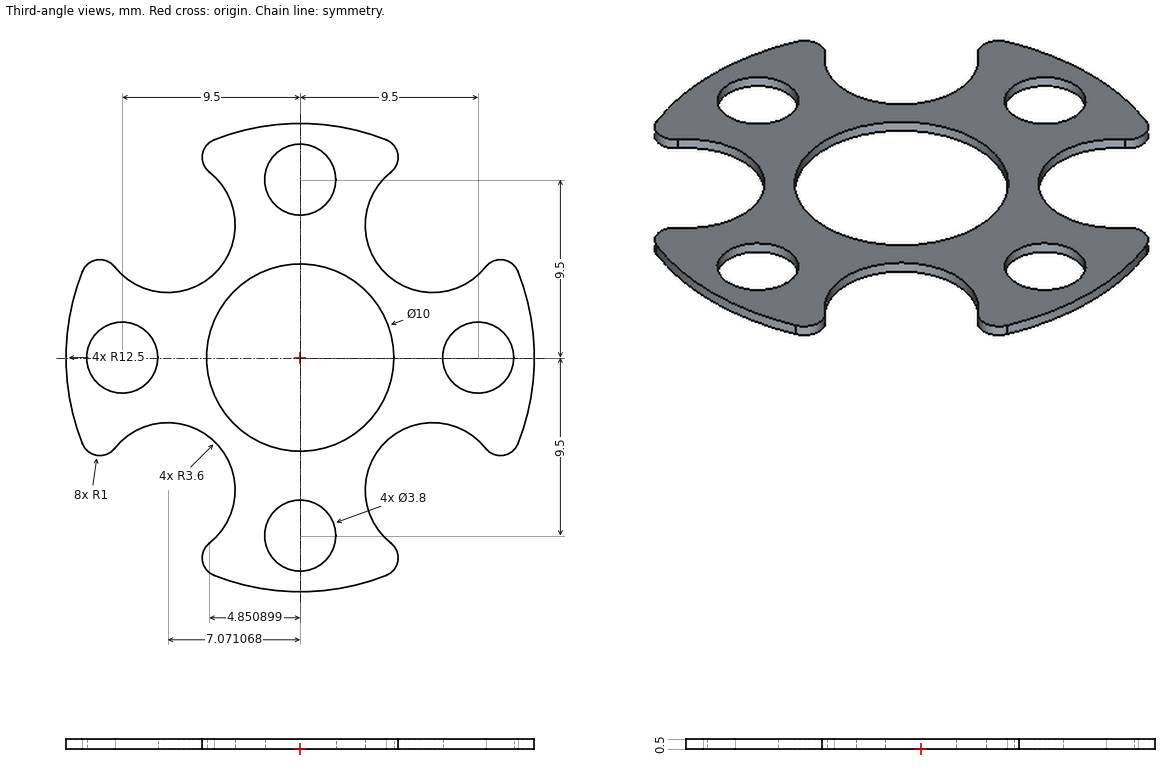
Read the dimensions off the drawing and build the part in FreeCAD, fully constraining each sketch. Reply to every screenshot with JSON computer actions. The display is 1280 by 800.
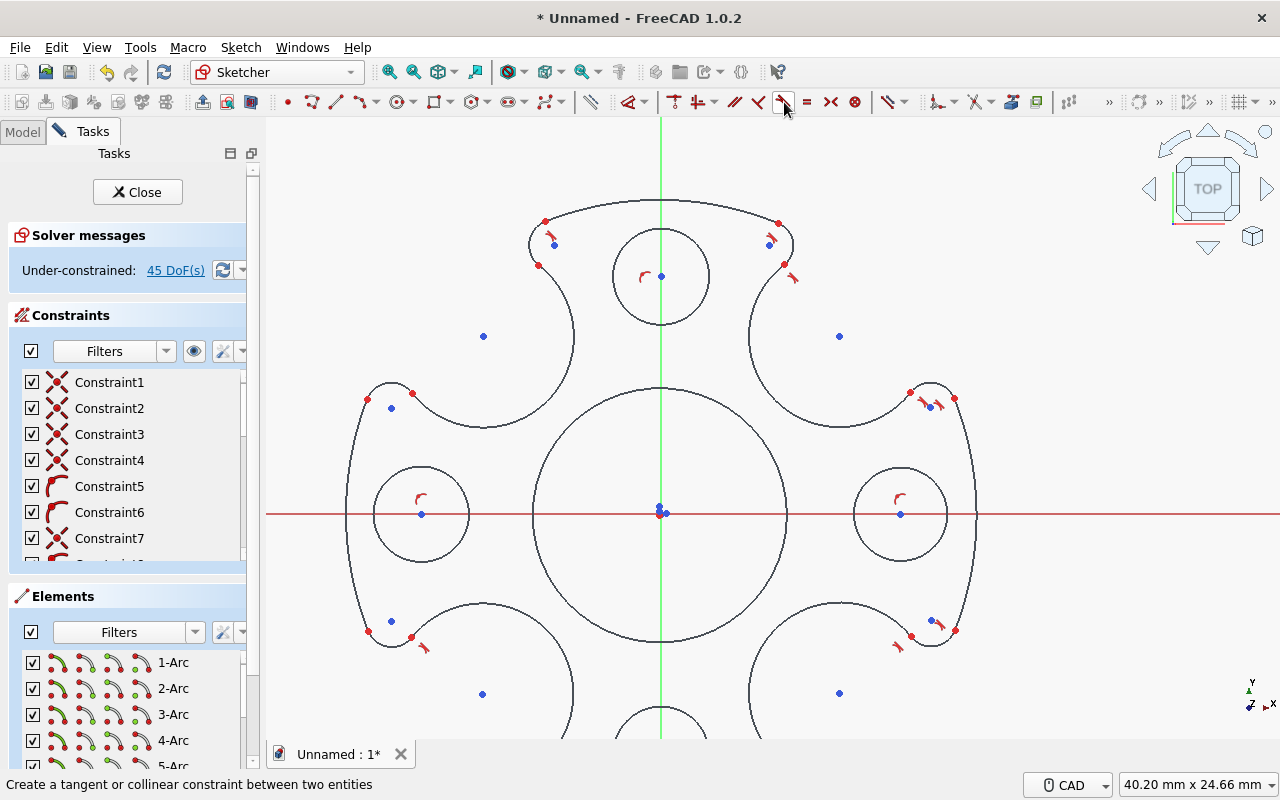
{"action": "left_click", "coordinate": [533, 231]}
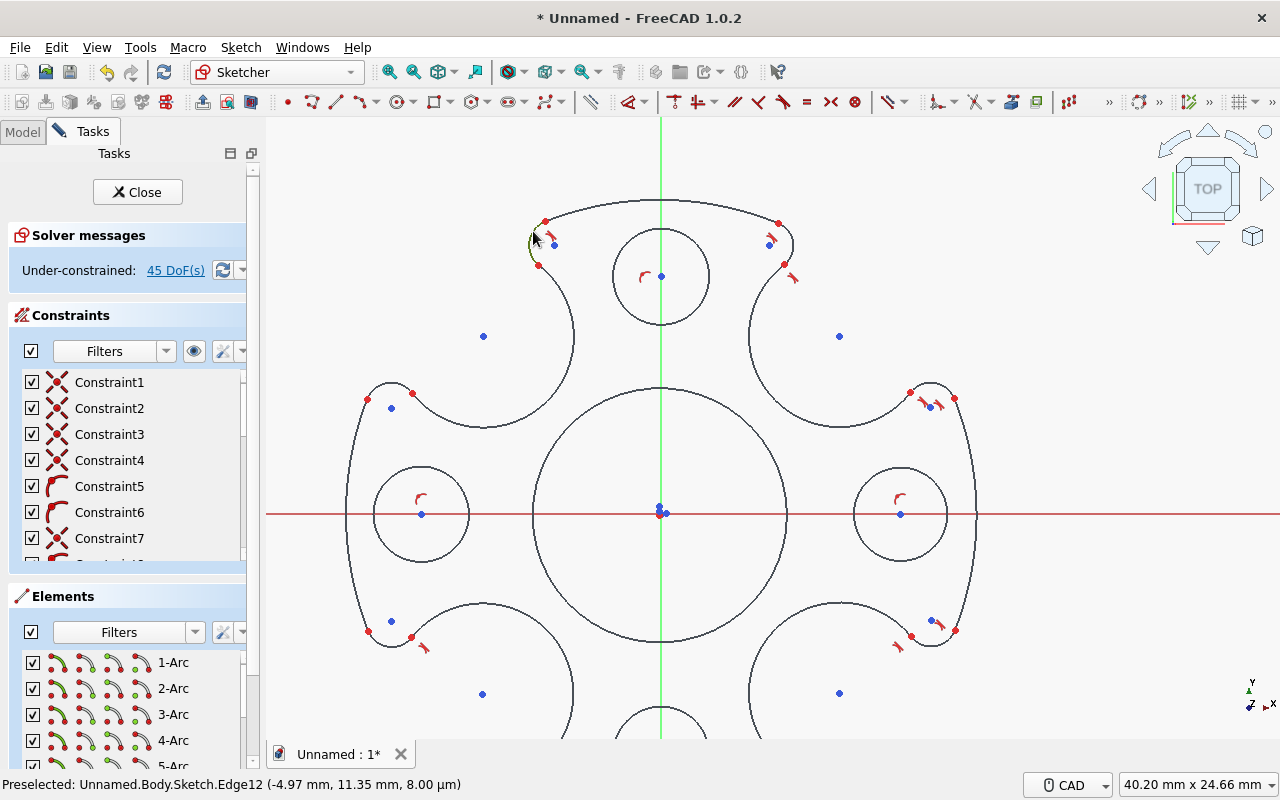
{"action": "left_click", "coordinate": [493, 427]}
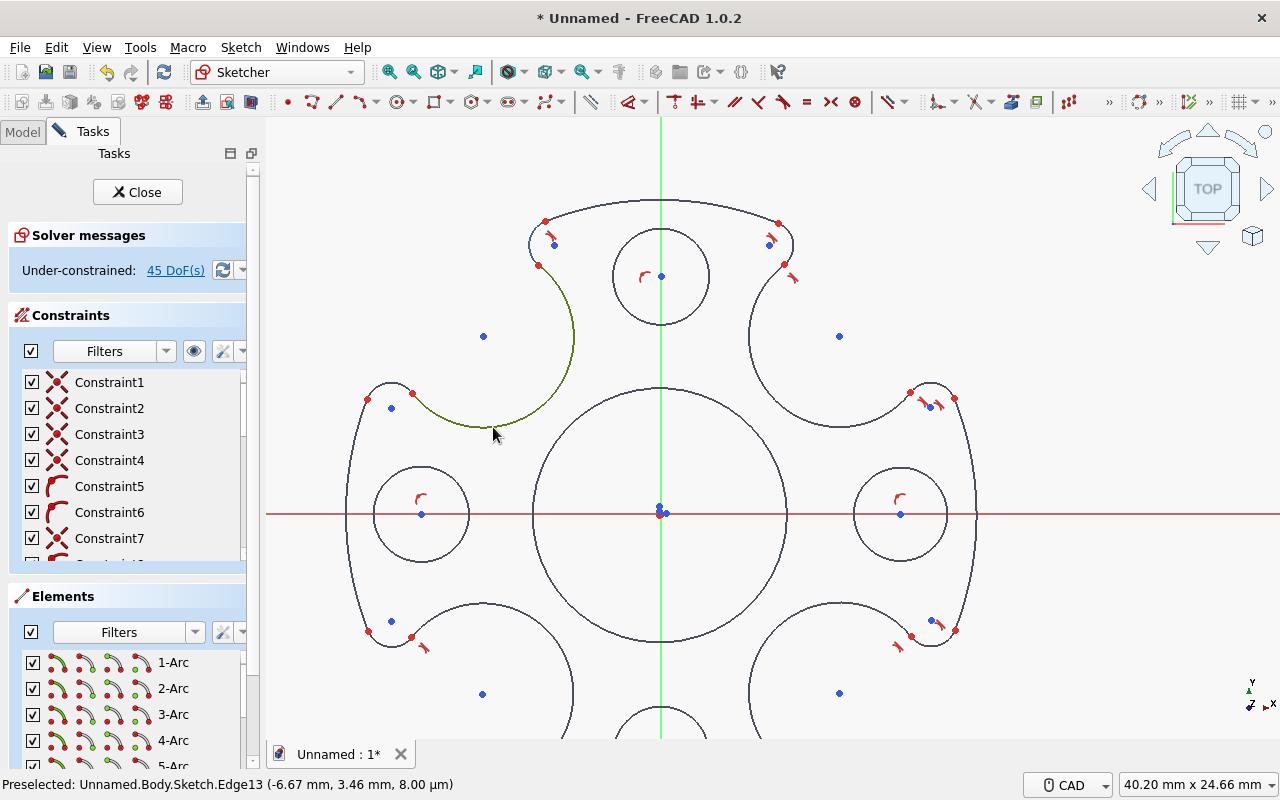
{"action": "key", "text": "t"}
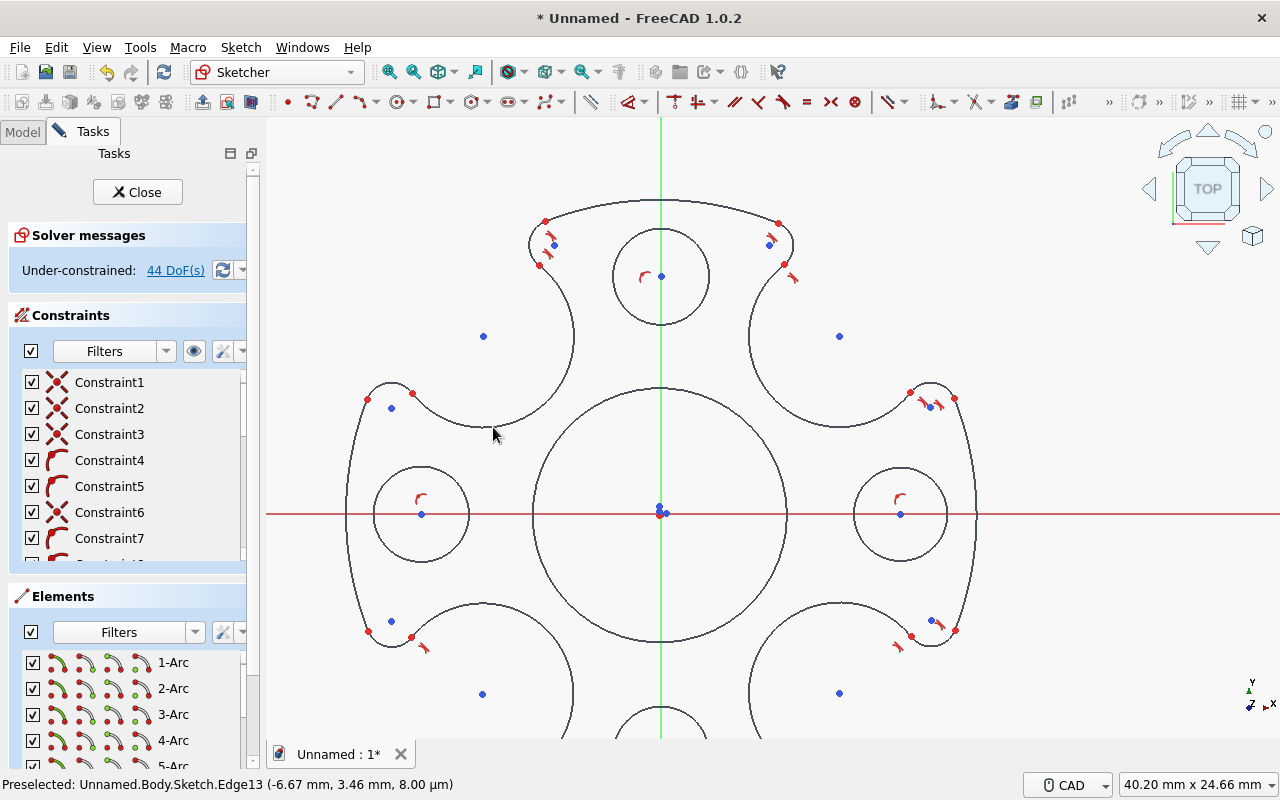
{"action": "left_click", "coordinate": [493, 427]}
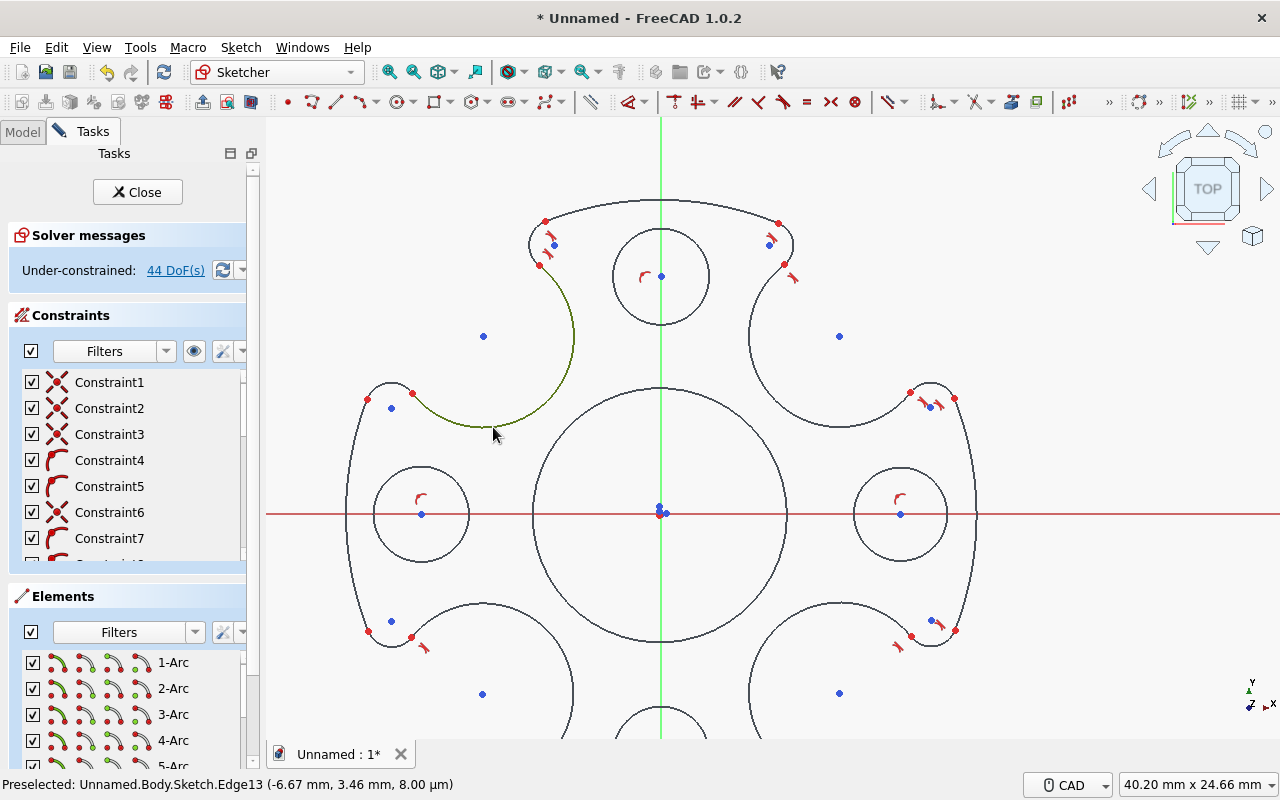
{"action": "left_click", "coordinate": [399, 384]}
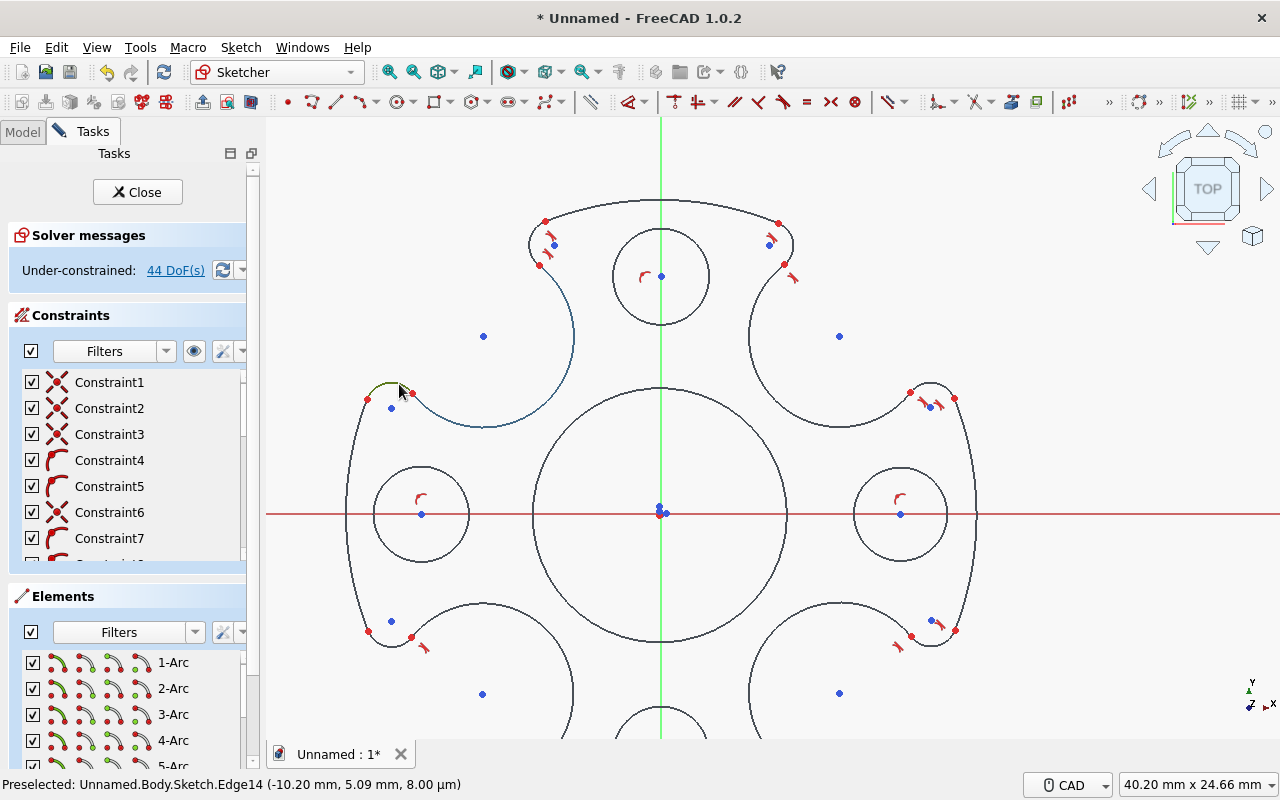
{"action": "left_click", "coordinate": [784, 102]}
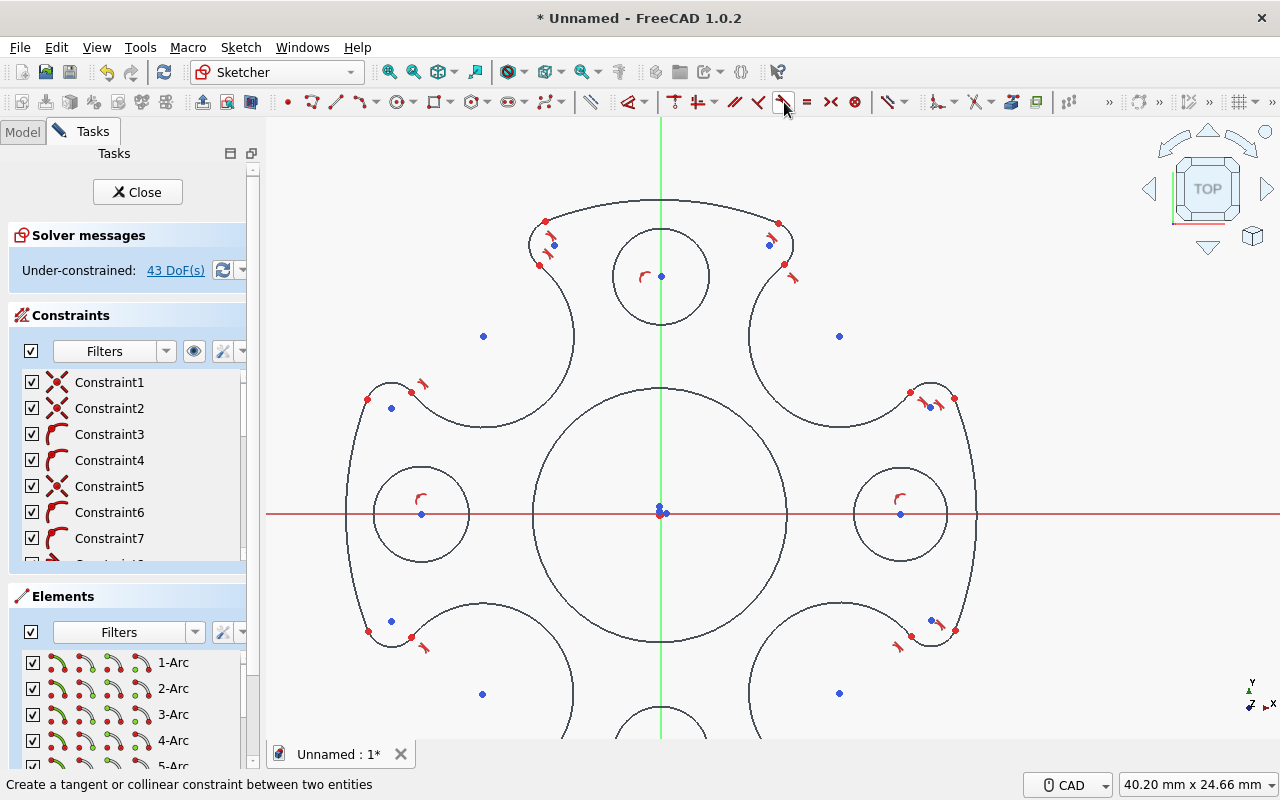
{"action": "left_click", "coordinate": [398, 384]}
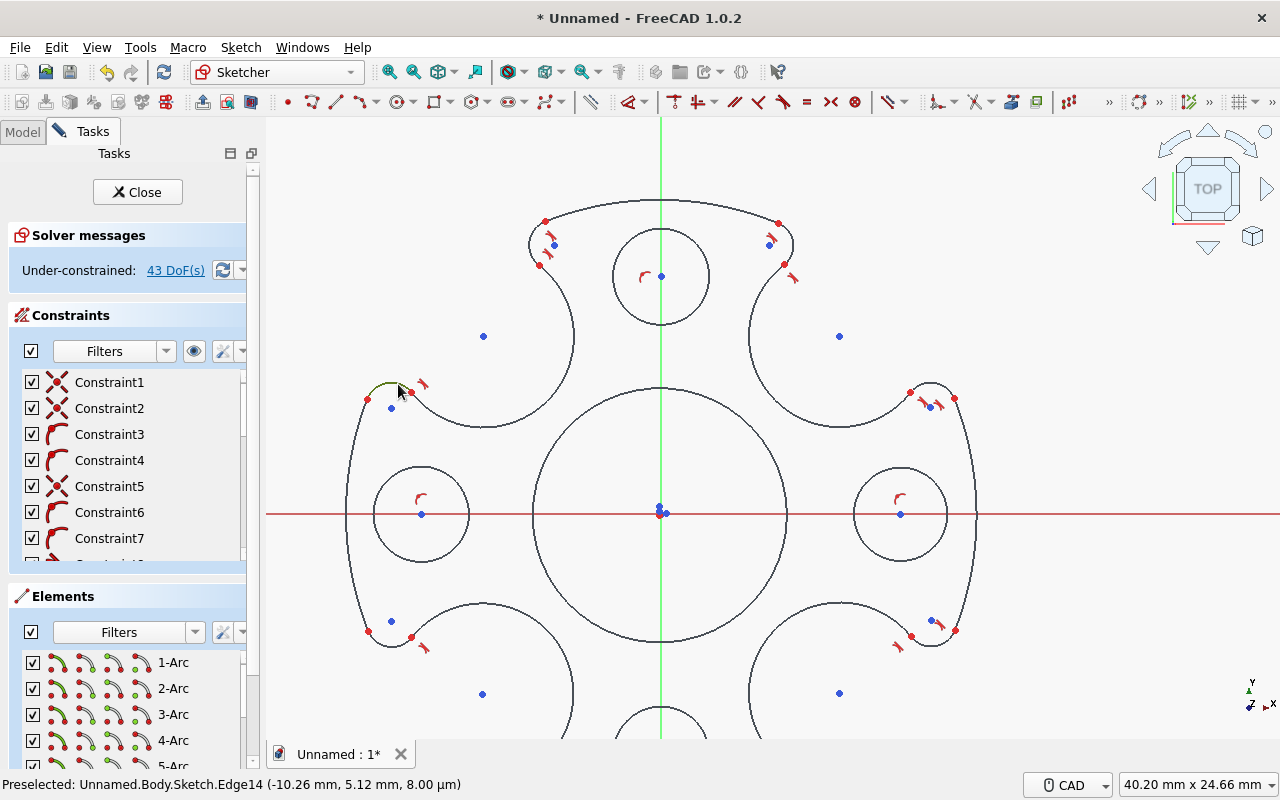
{"action": "left_click", "coordinate": [349, 468]}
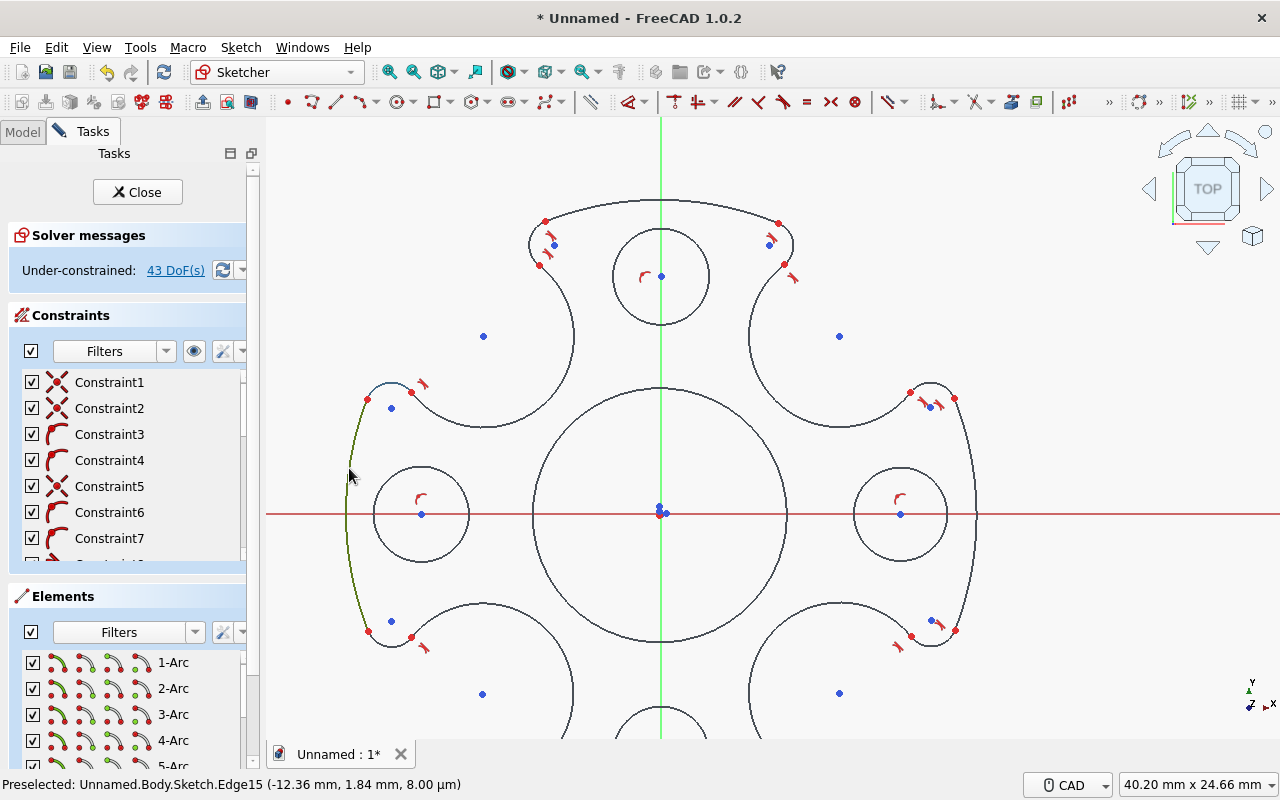
{"action": "key", "text": "t"}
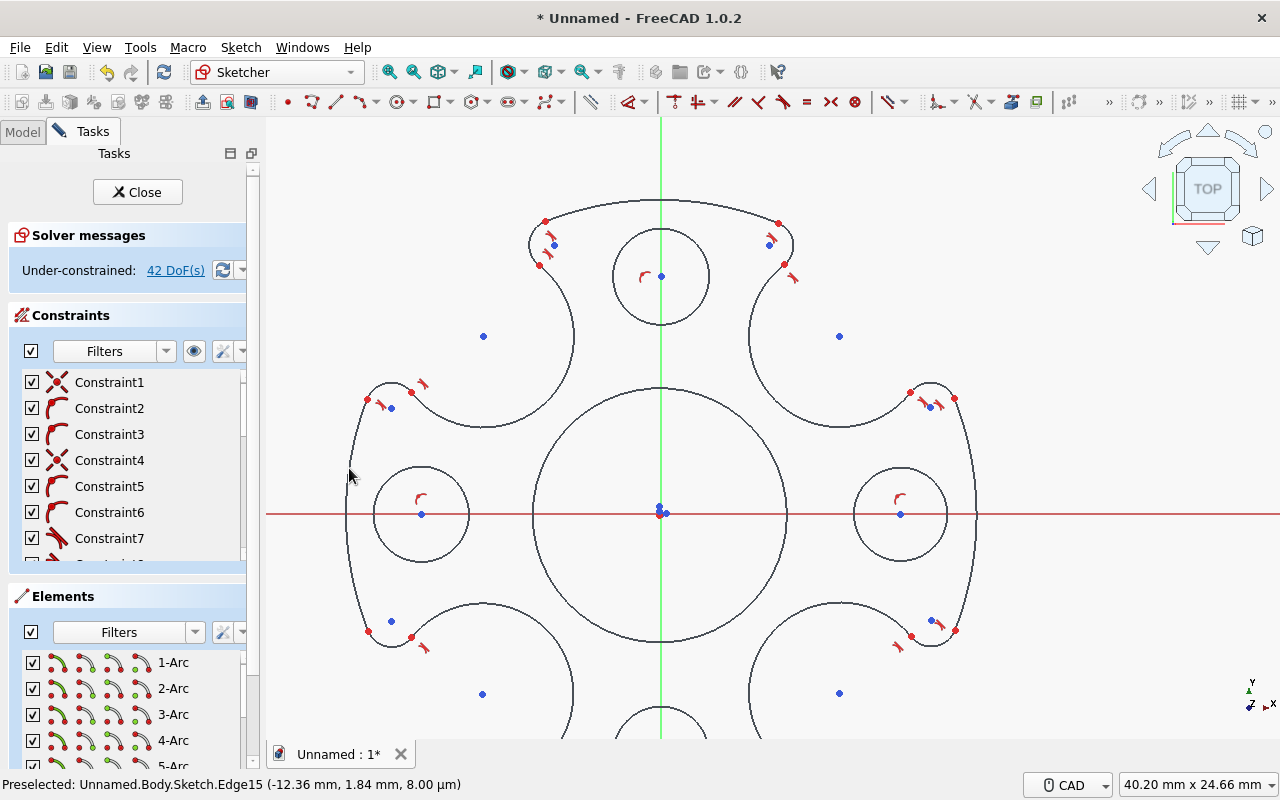
{"action": "left_click", "coordinate": [349, 468]}